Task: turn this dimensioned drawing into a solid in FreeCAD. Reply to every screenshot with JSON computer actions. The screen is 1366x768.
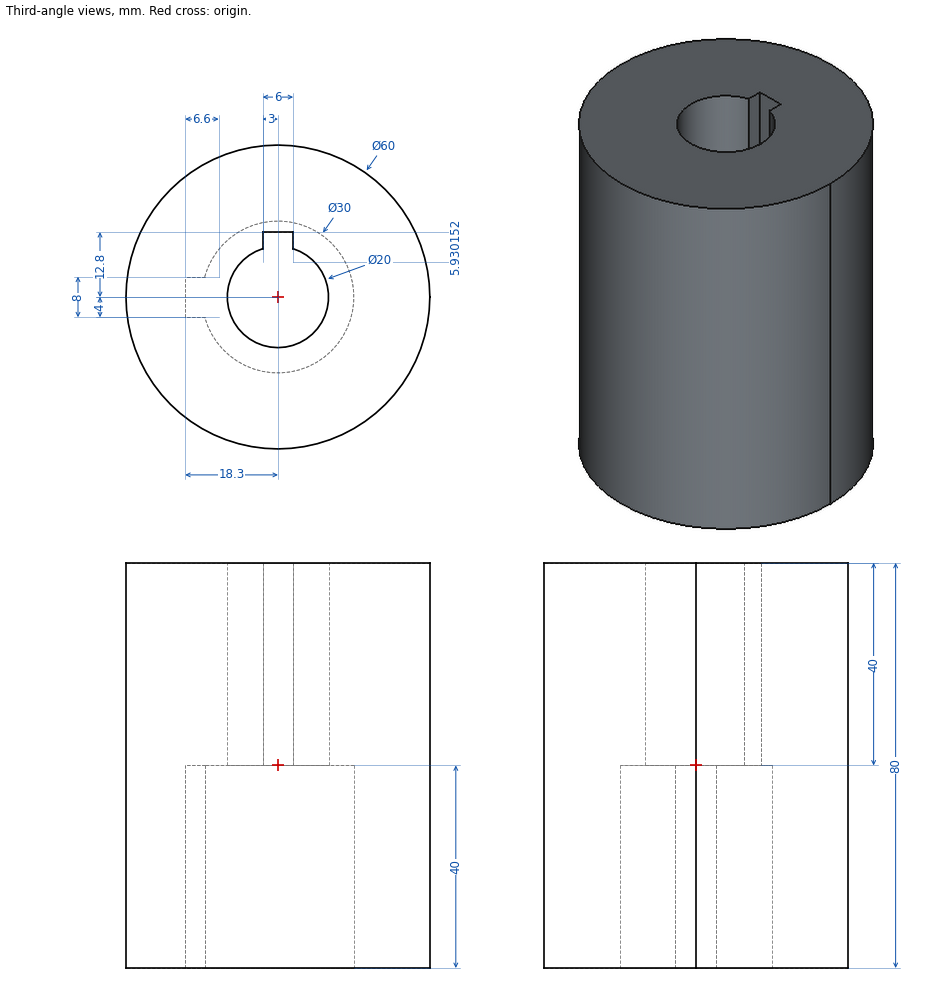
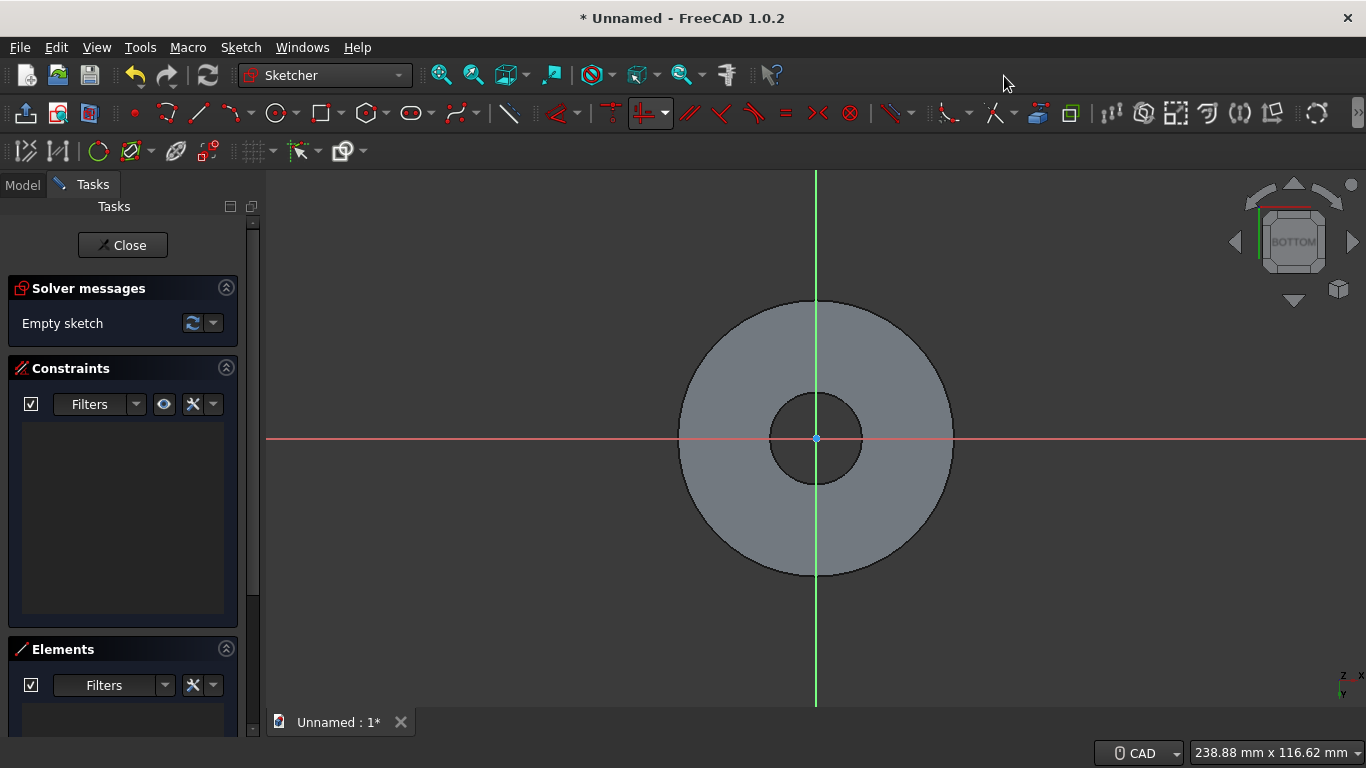
{"action": "scroll", "coordinate": [872, 438], "scroll_direction": "up", "scroll_amount": 4}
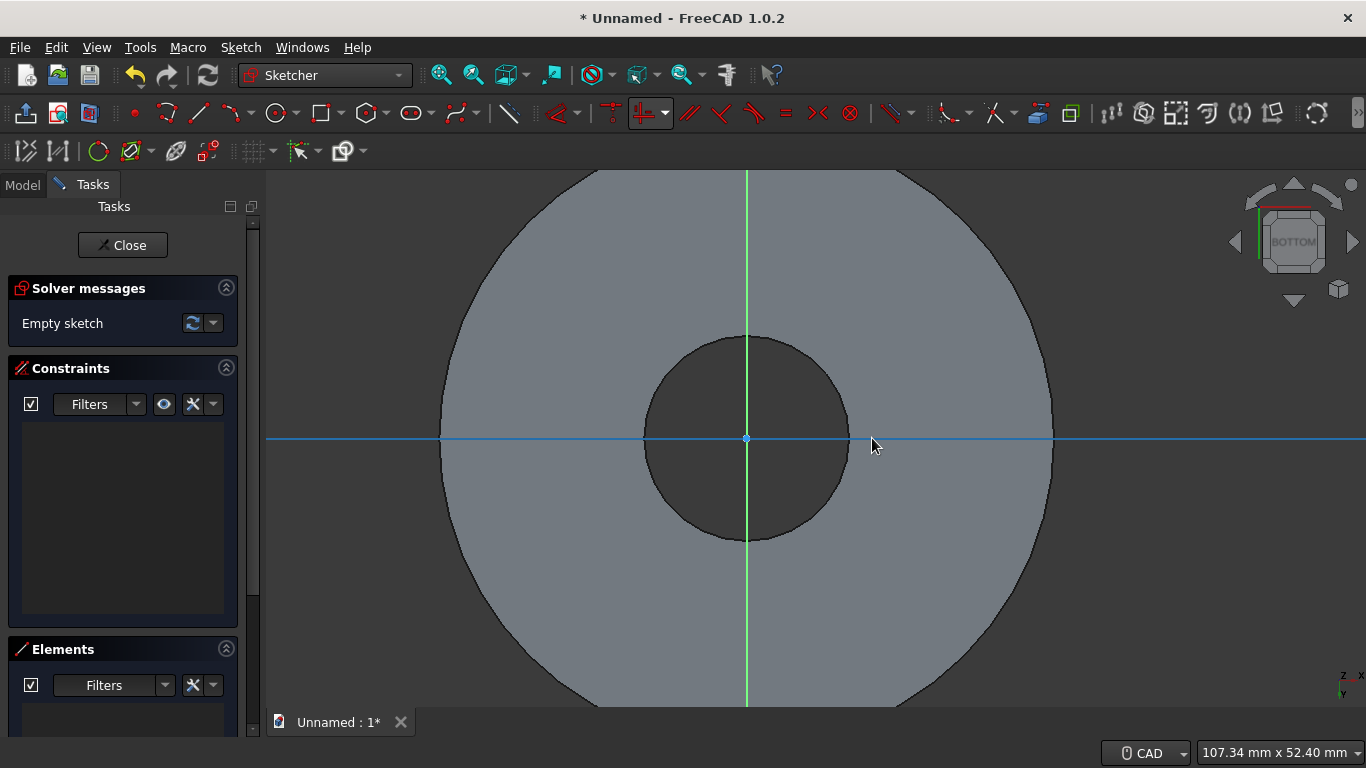
{"action": "key", "text": "g c"}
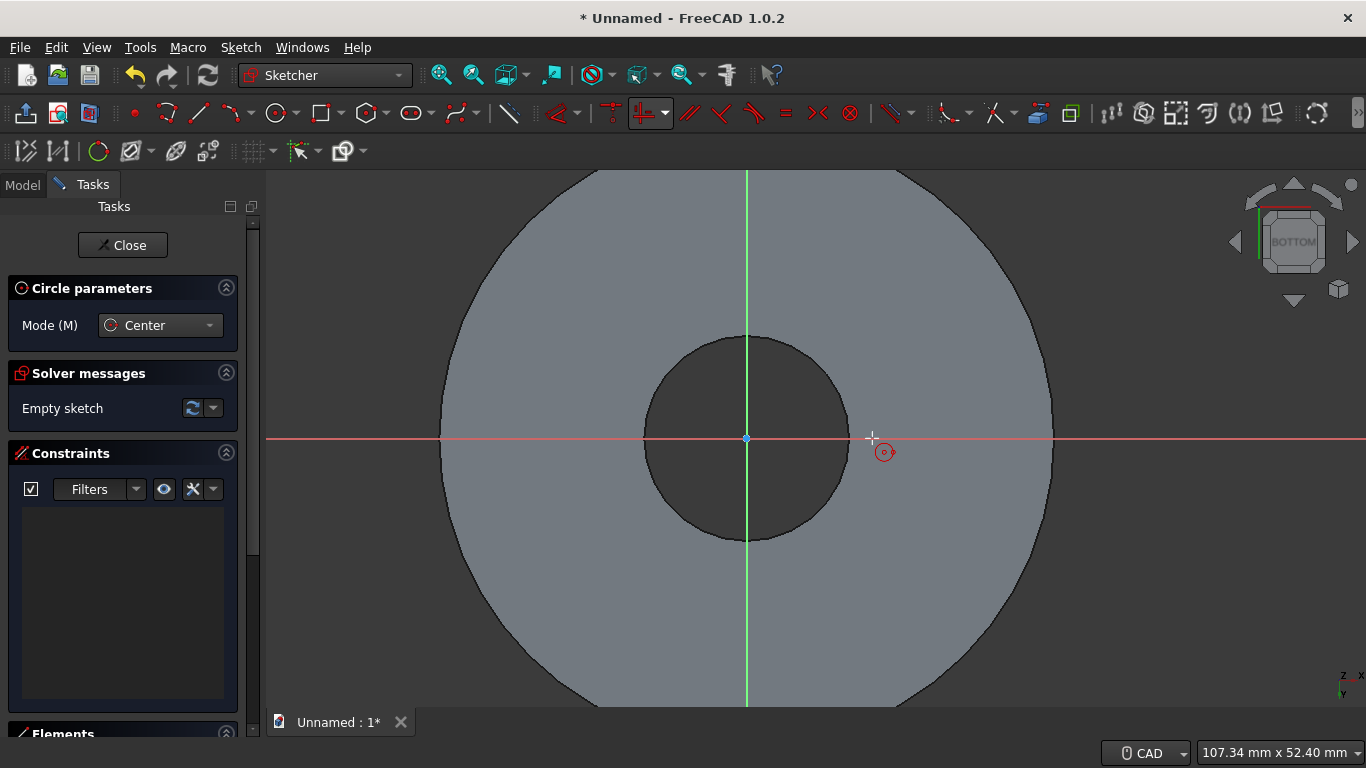
{"action": "left_click", "coordinate": [747, 438]}
{"action": "mouse_move", "coordinate": [855, 330]}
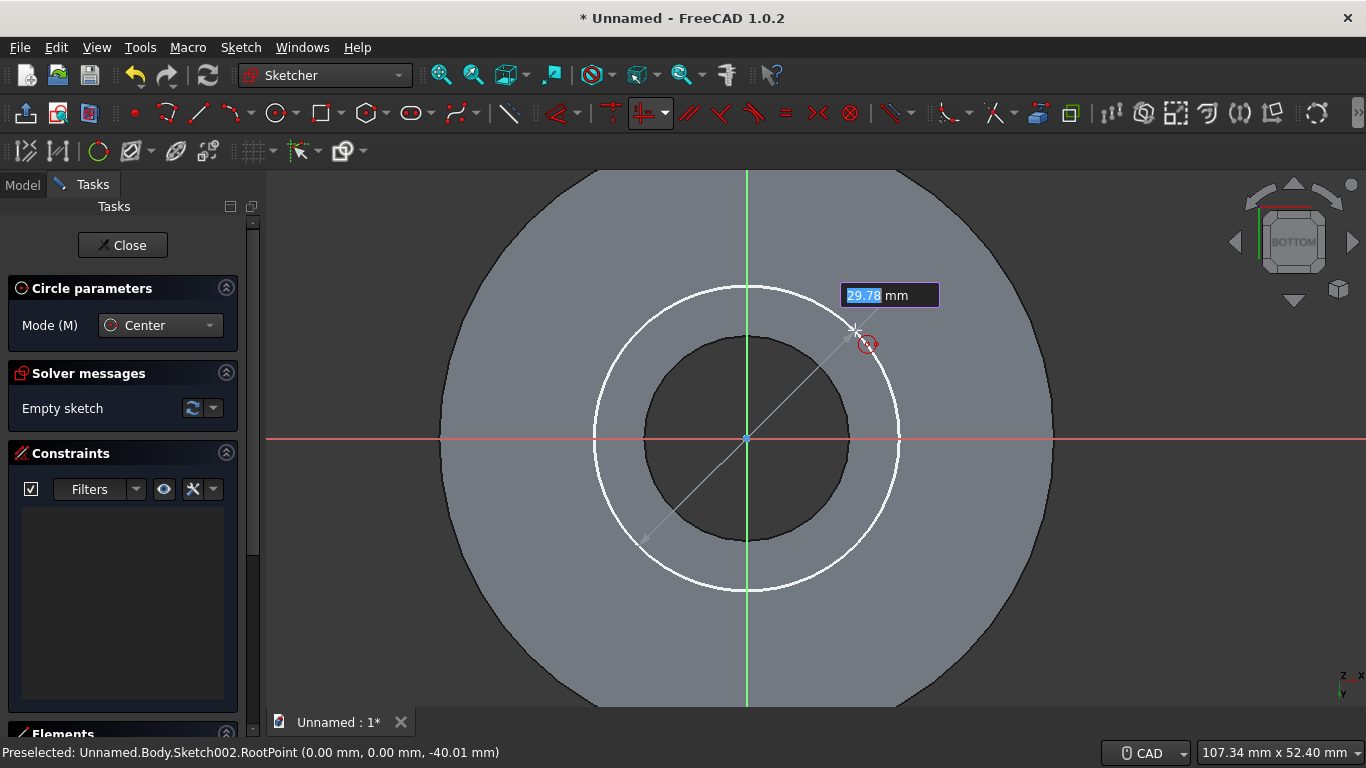
{"action": "type", "text": "30"}
{"action": "key", "text": "Return"}
{"action": "key", "text": "Escape"}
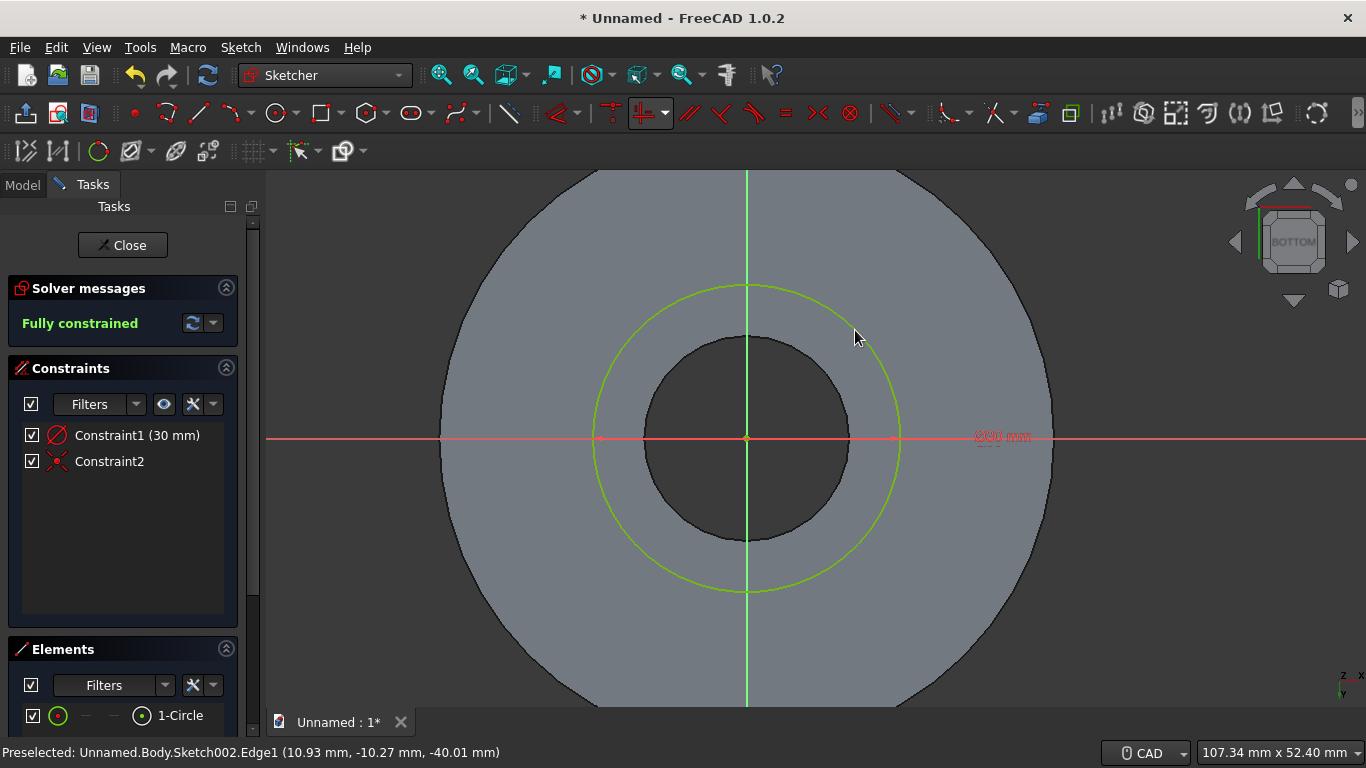
{"action": "left_click", "coordinate": [123, 245]}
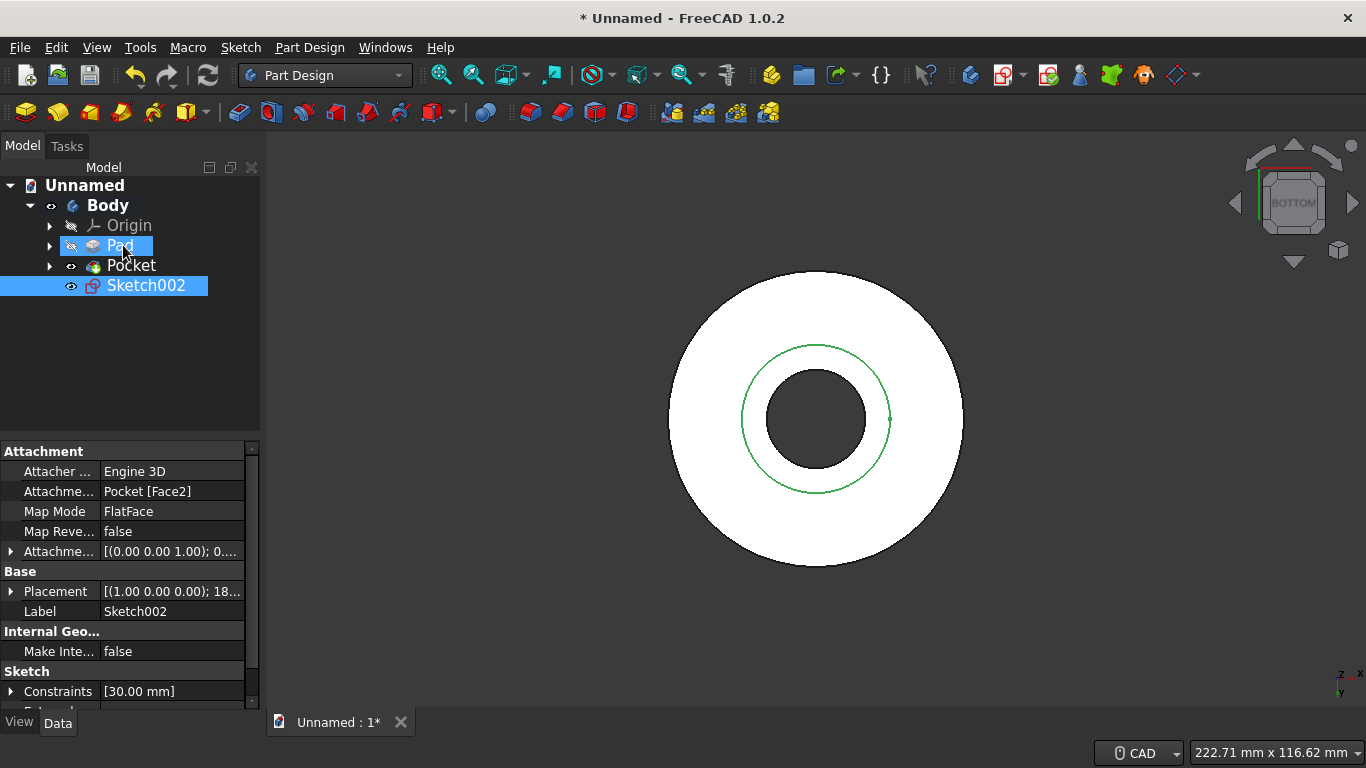
{"action": "left_click", "coordinate": [240, 112]}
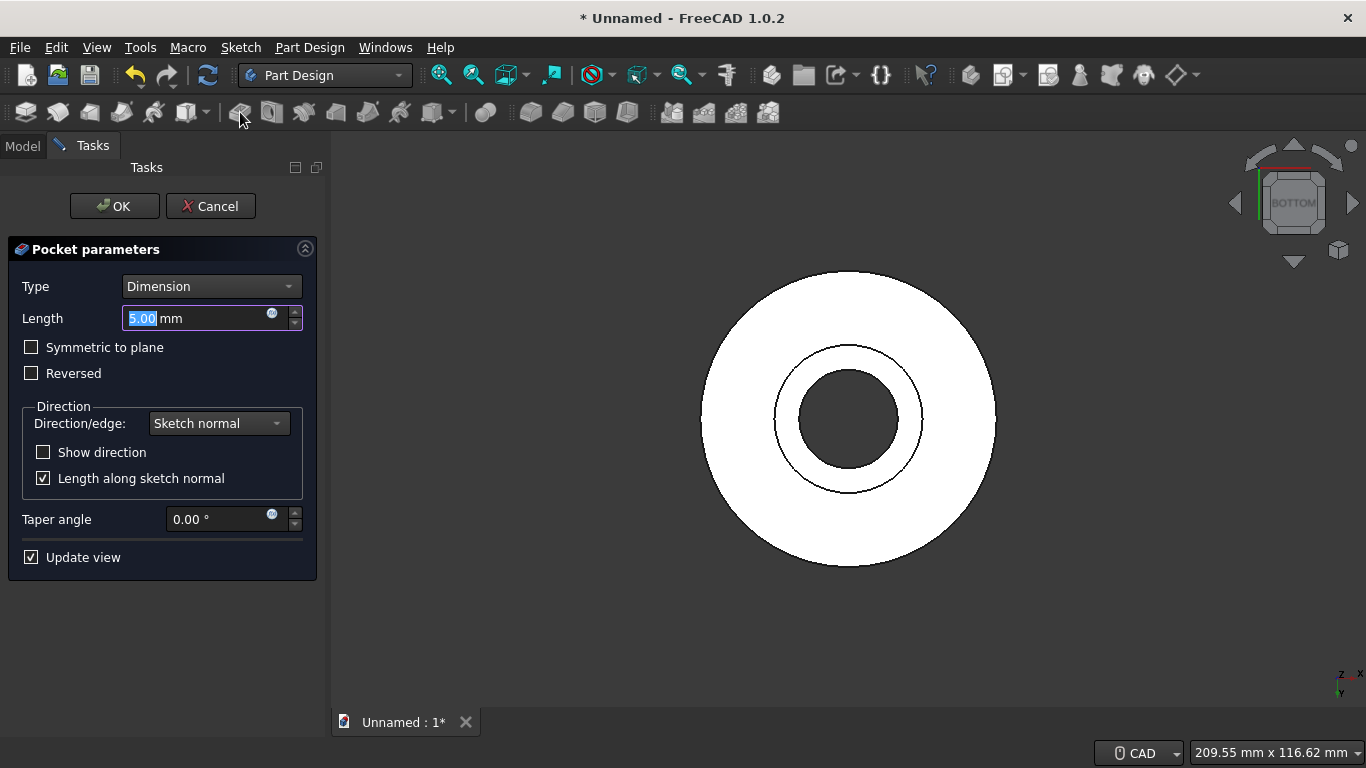
{"action": "type", "text": "40"}
{"action": "key", "text": "Tab"}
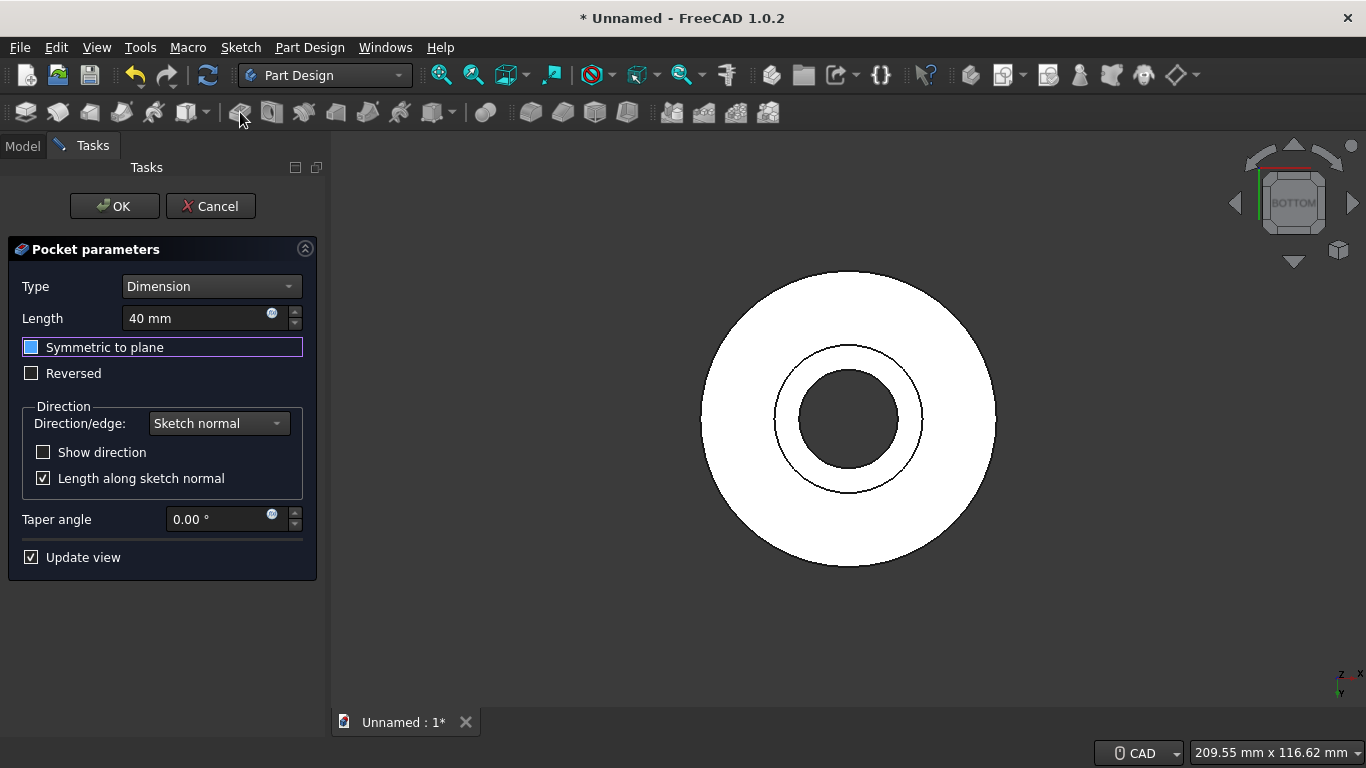
{"action": "left_click", "coordinate": [115, 206]}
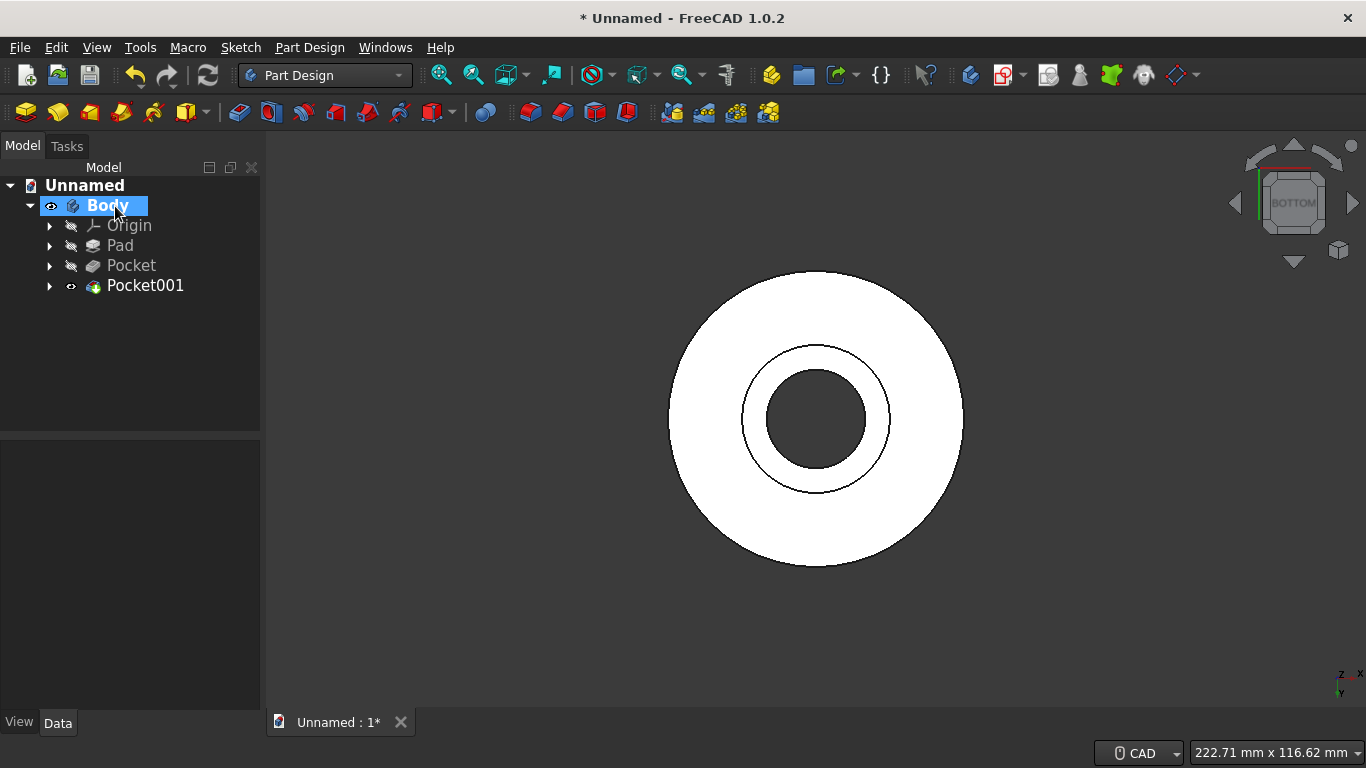
{"action": "key", "text": "0"}